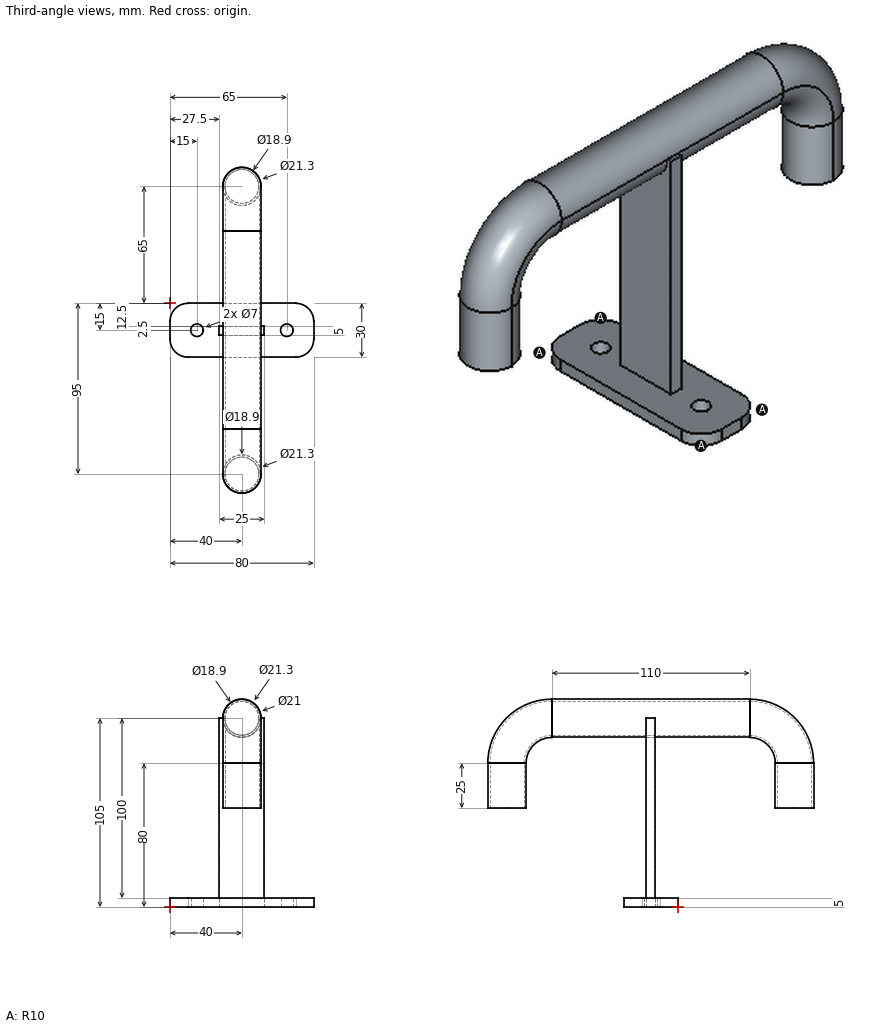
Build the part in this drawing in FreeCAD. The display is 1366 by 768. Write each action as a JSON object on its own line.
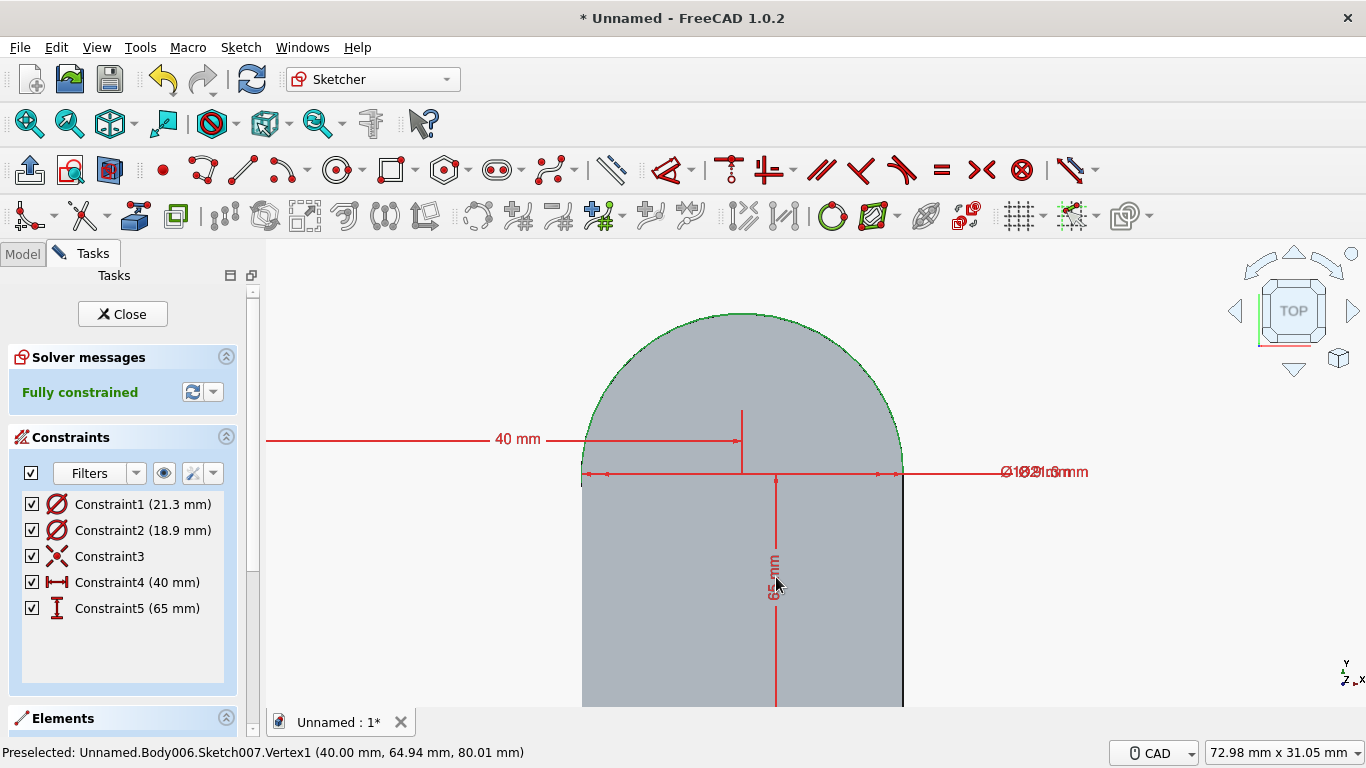
{"action": "left_click", "coordinate": [123, 314]}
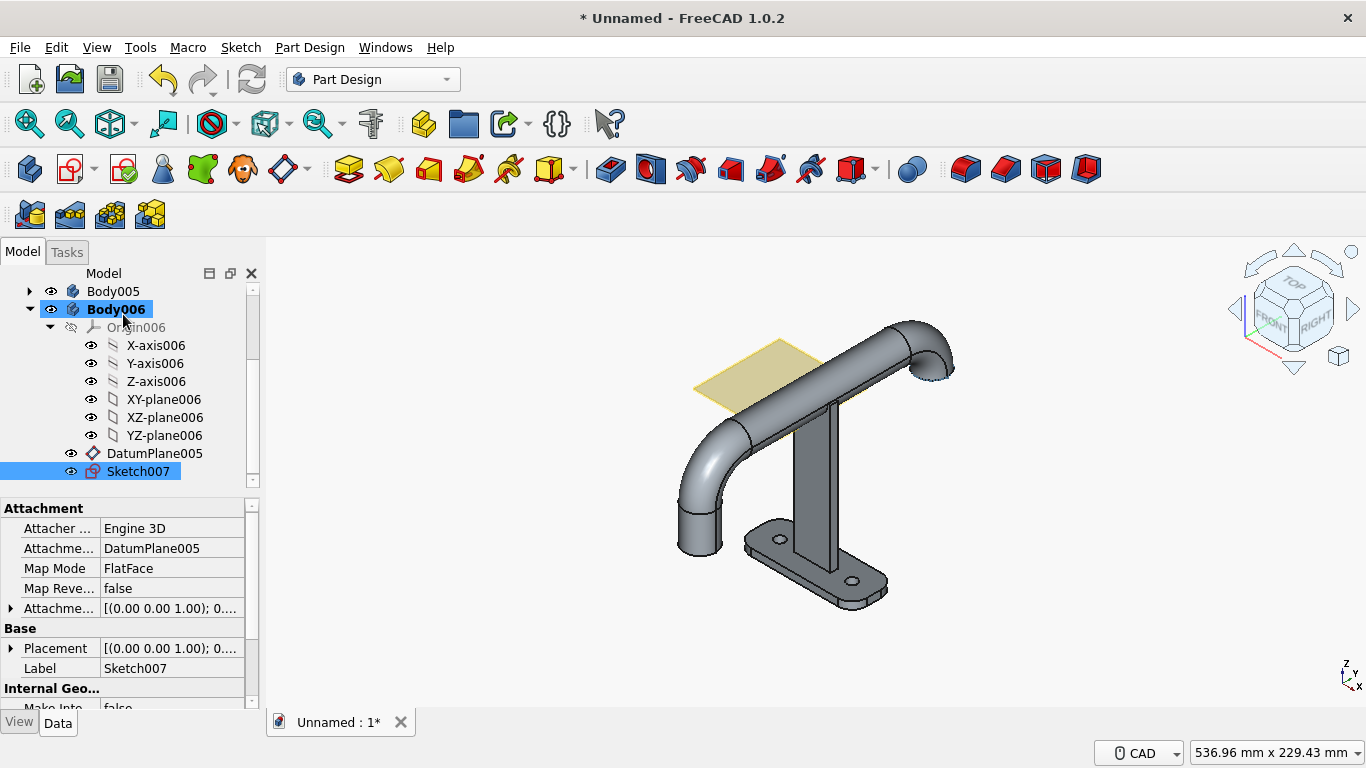
{"action": "left_click", "coordinate": [350, 170]}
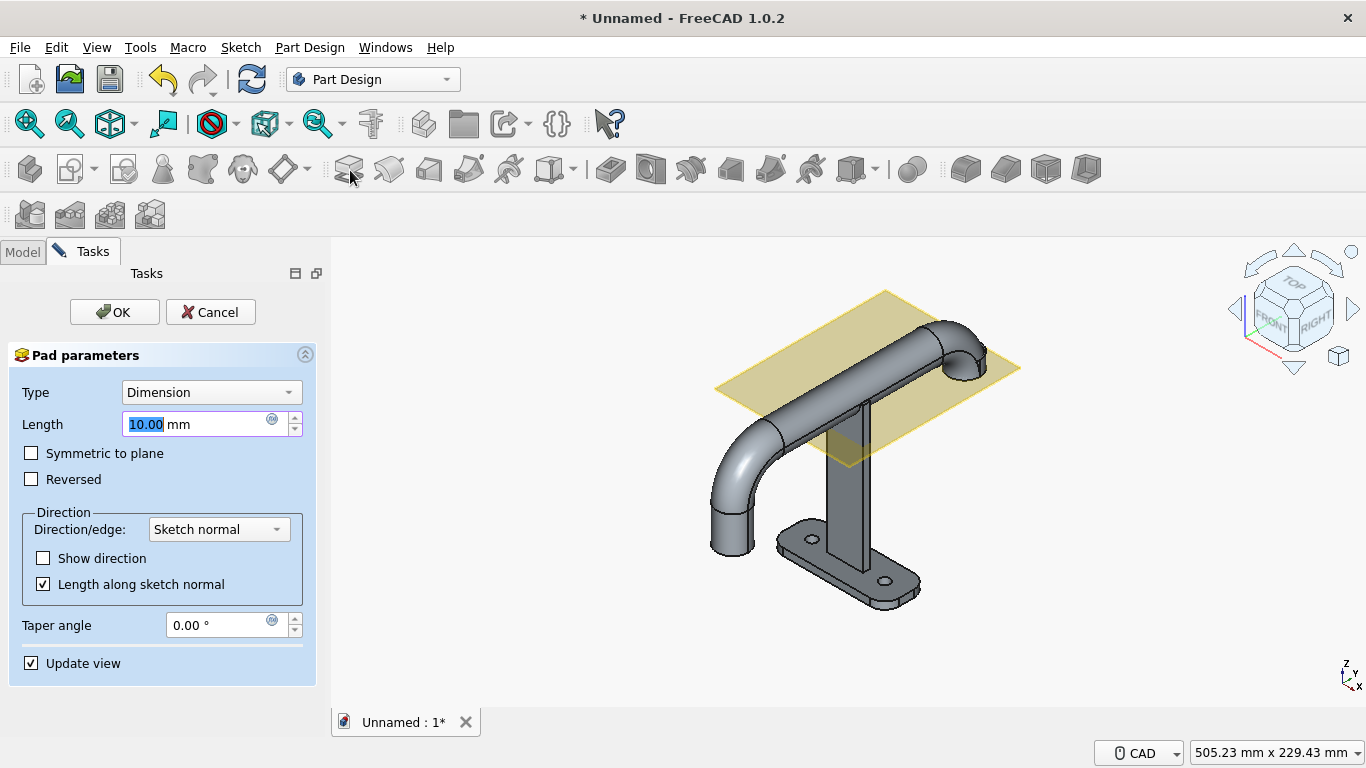
{"action": "type", "text": "25"}
{"action": "key", "text": "Tab"}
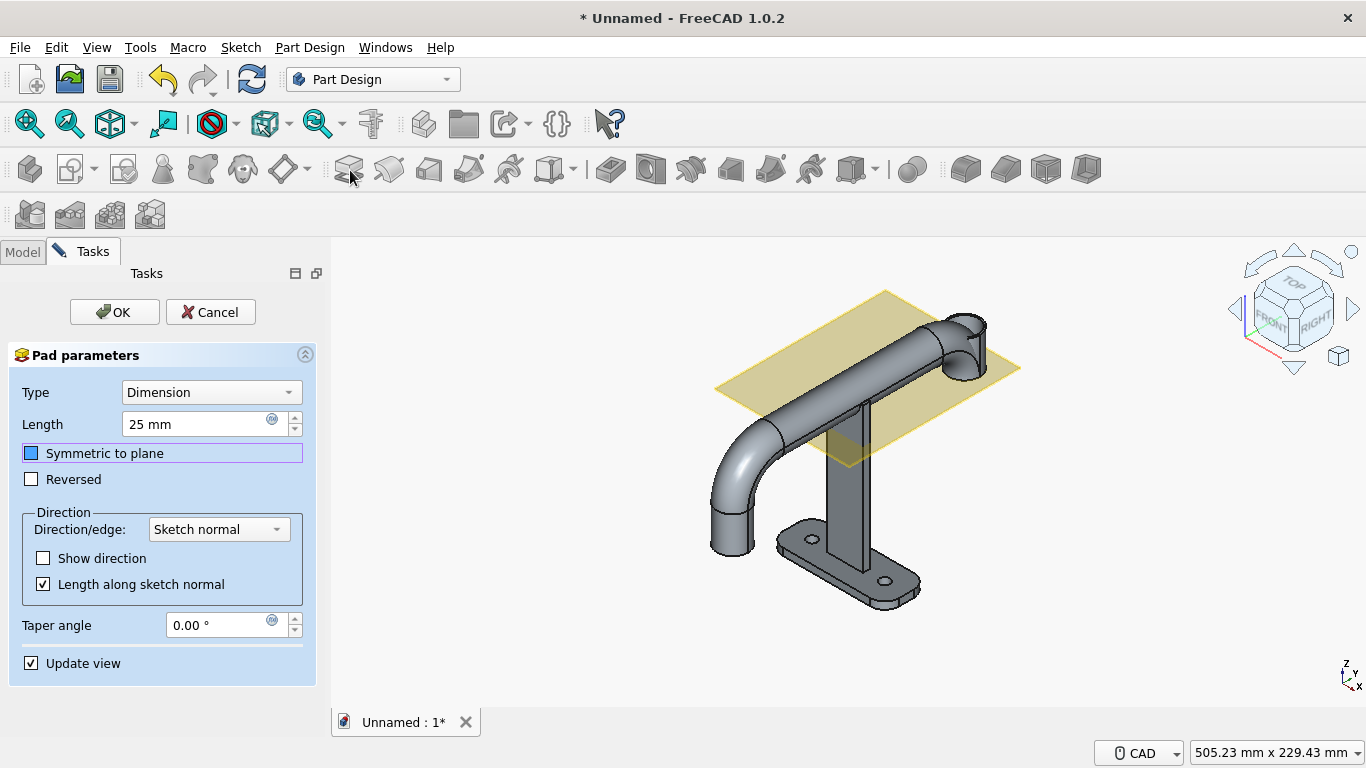
{"action": "left_click", "coordinate": [30, 479]}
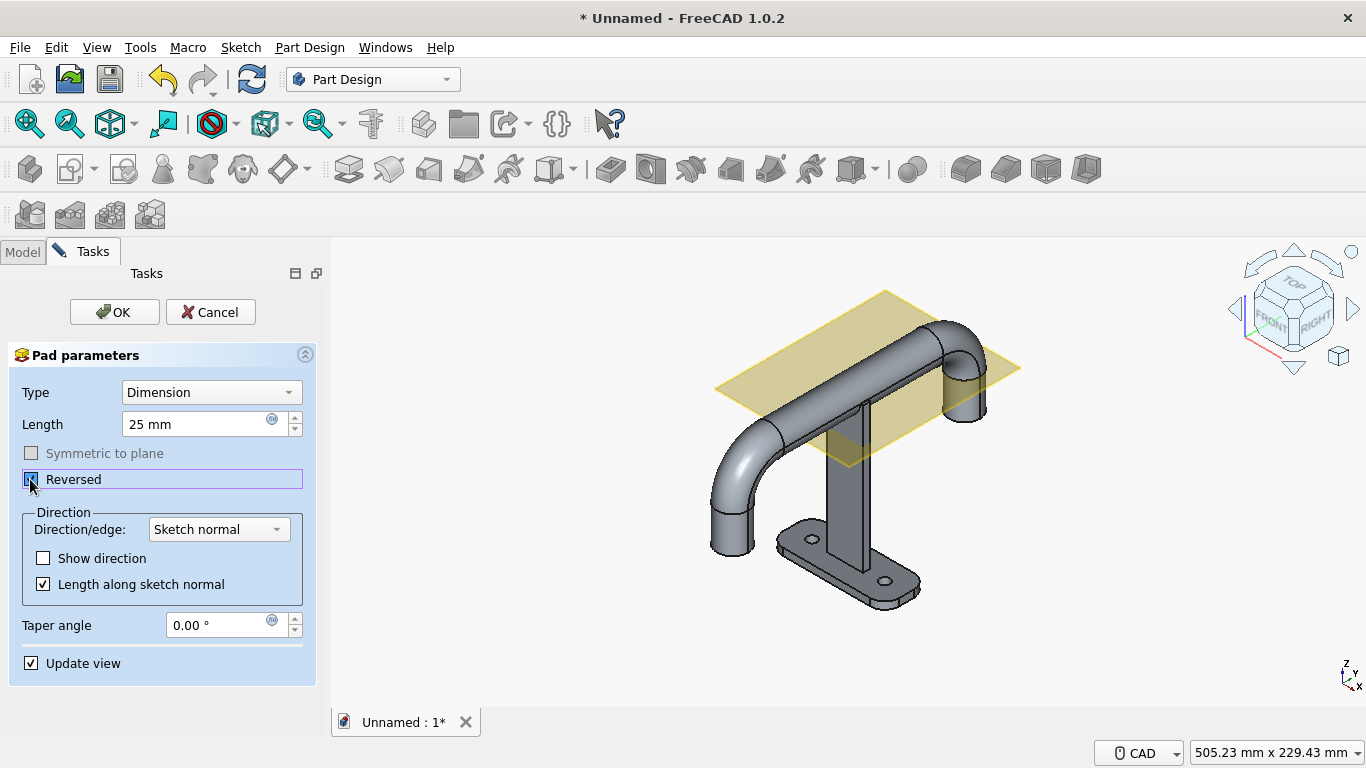
{"action": "left_click", "coordinate": [115, 312]}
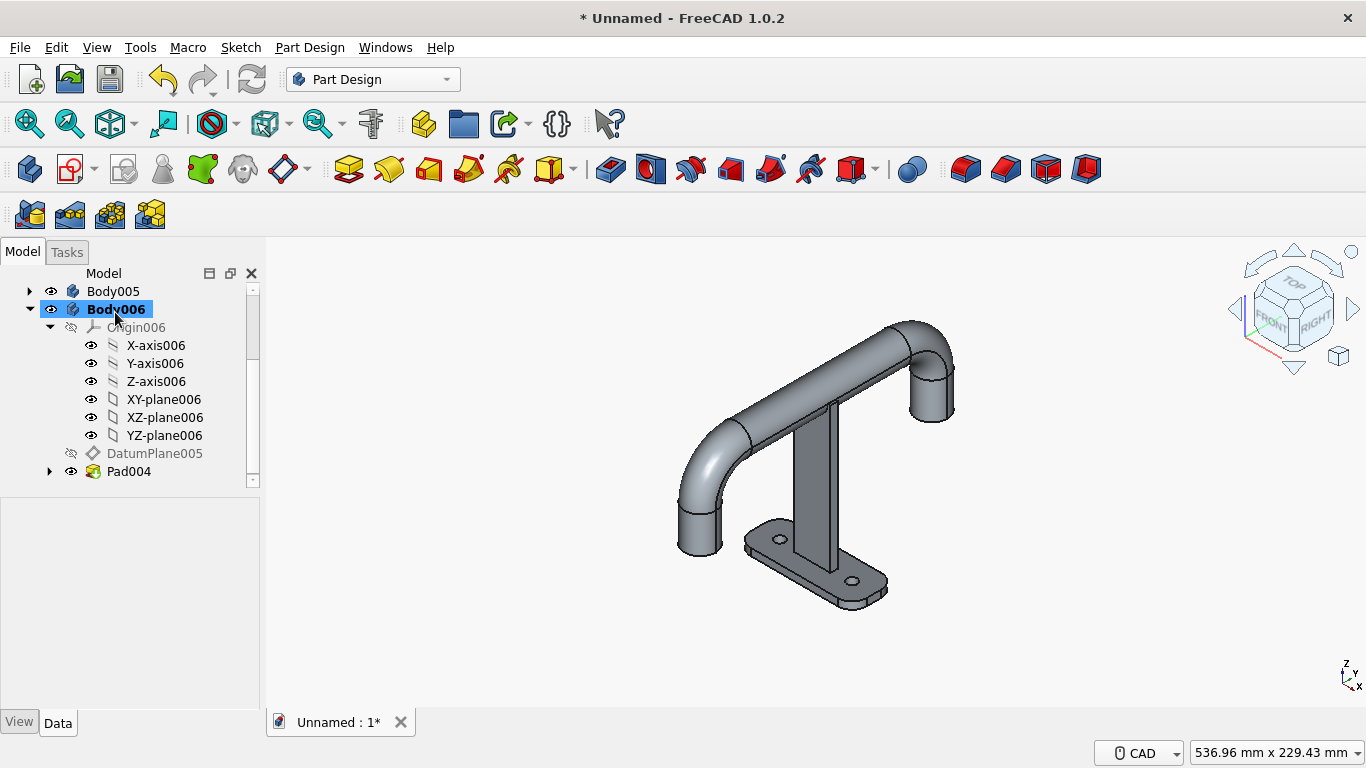
{"action": "left_click", "coordinate": [30, 124]}